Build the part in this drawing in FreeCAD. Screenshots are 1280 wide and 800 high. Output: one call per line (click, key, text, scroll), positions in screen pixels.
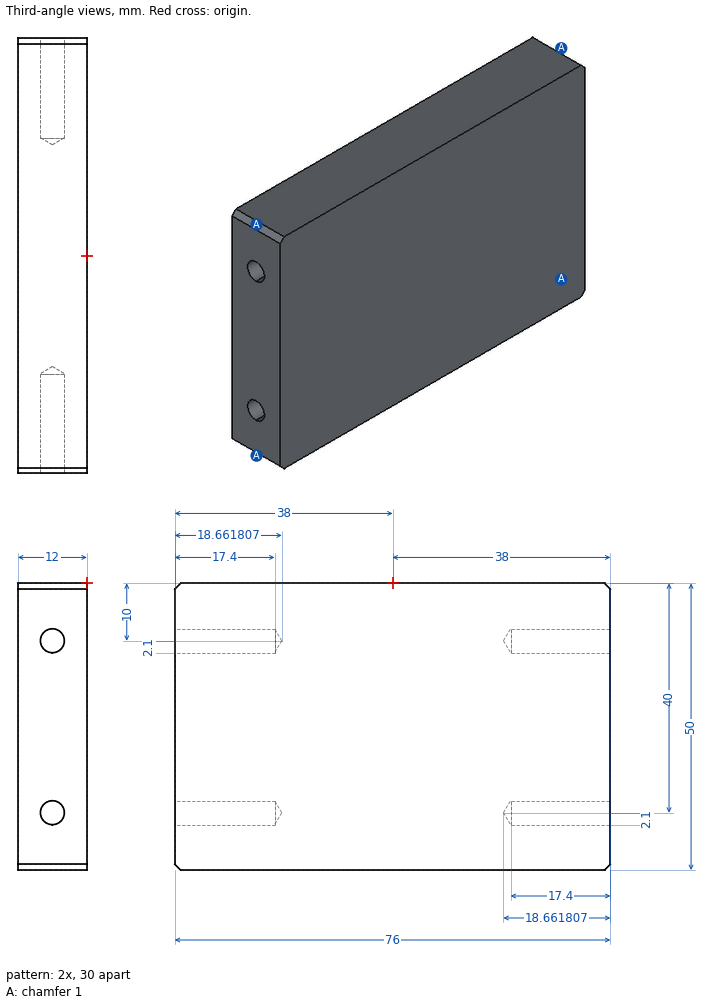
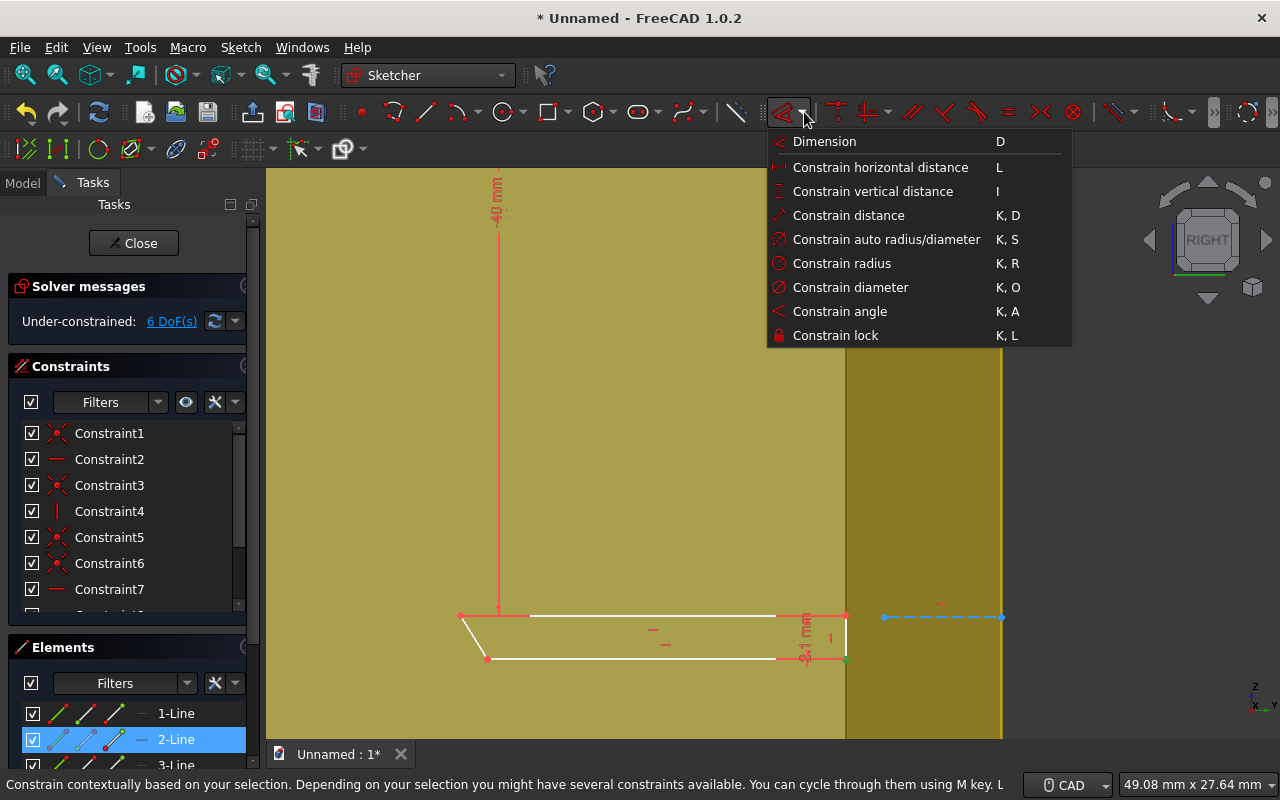
click(920, 167)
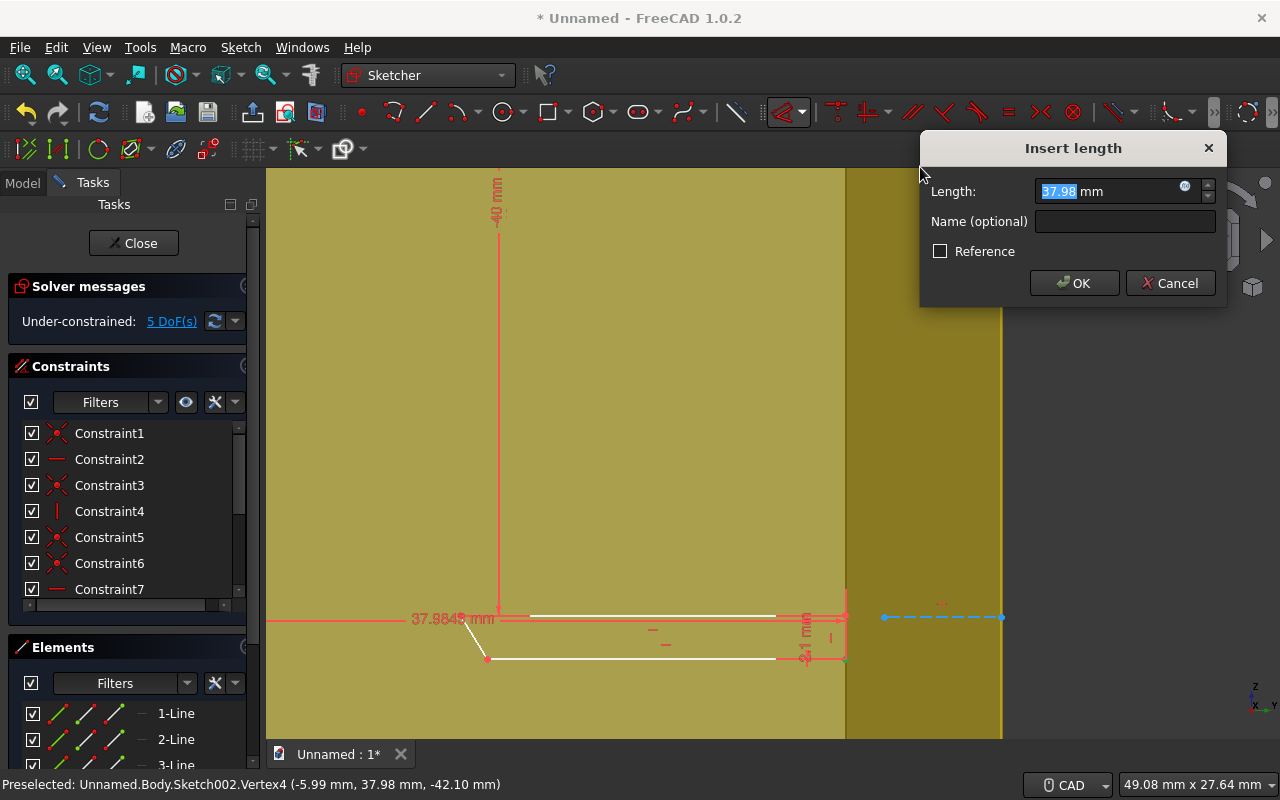
text(38)
key(Return)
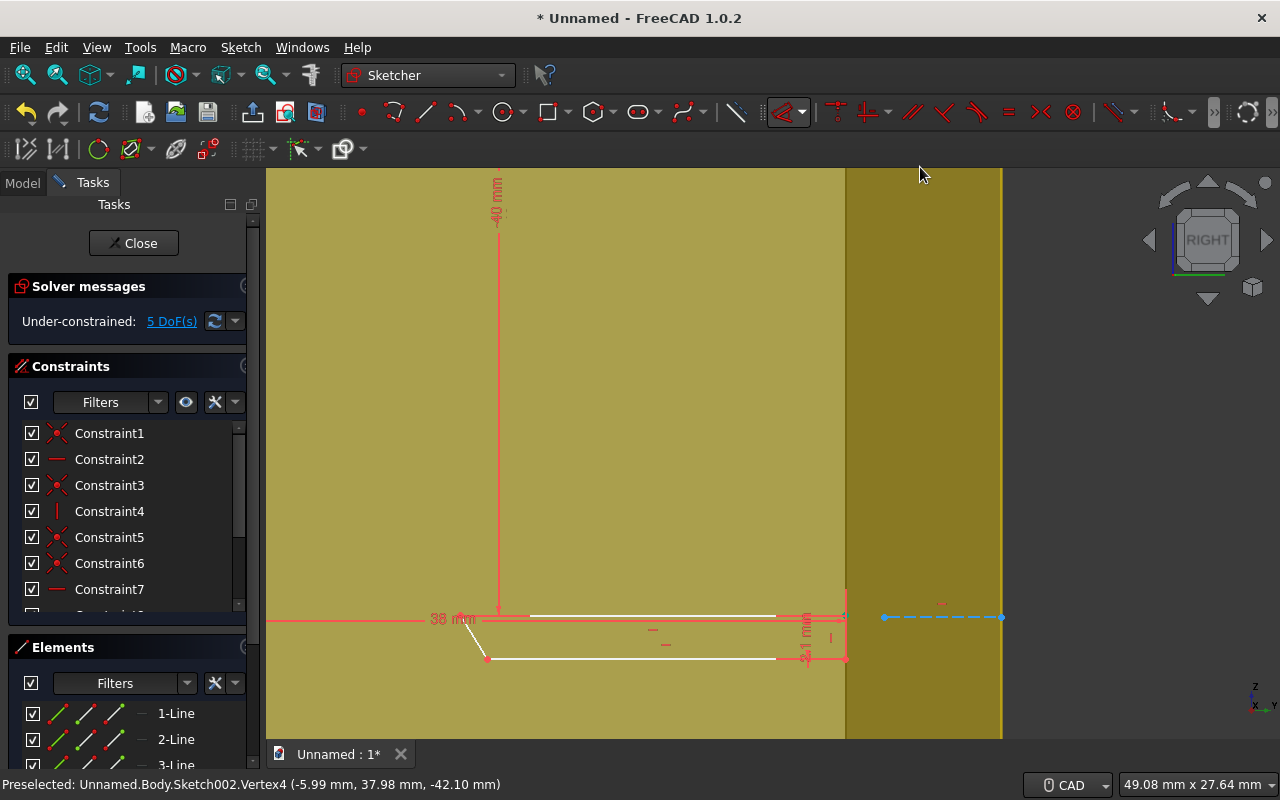
click(885, 617)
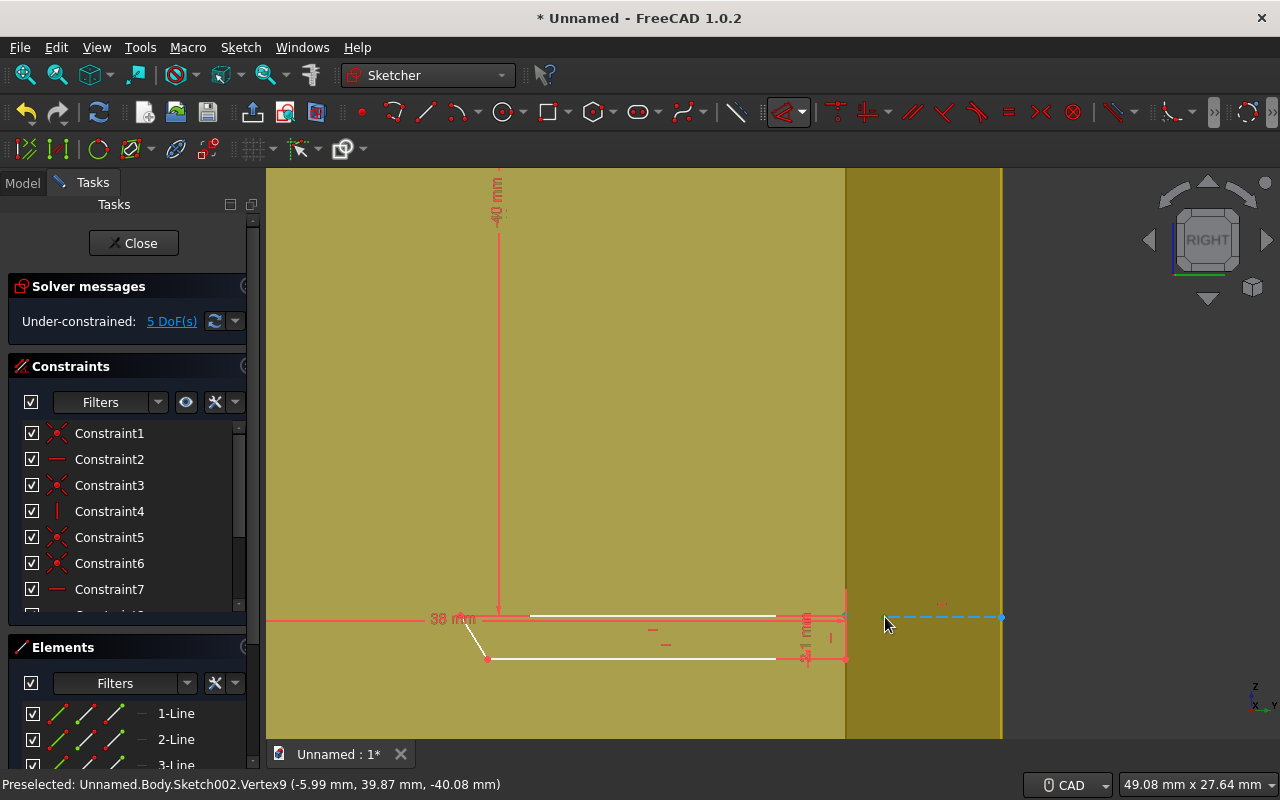
click(804, 112)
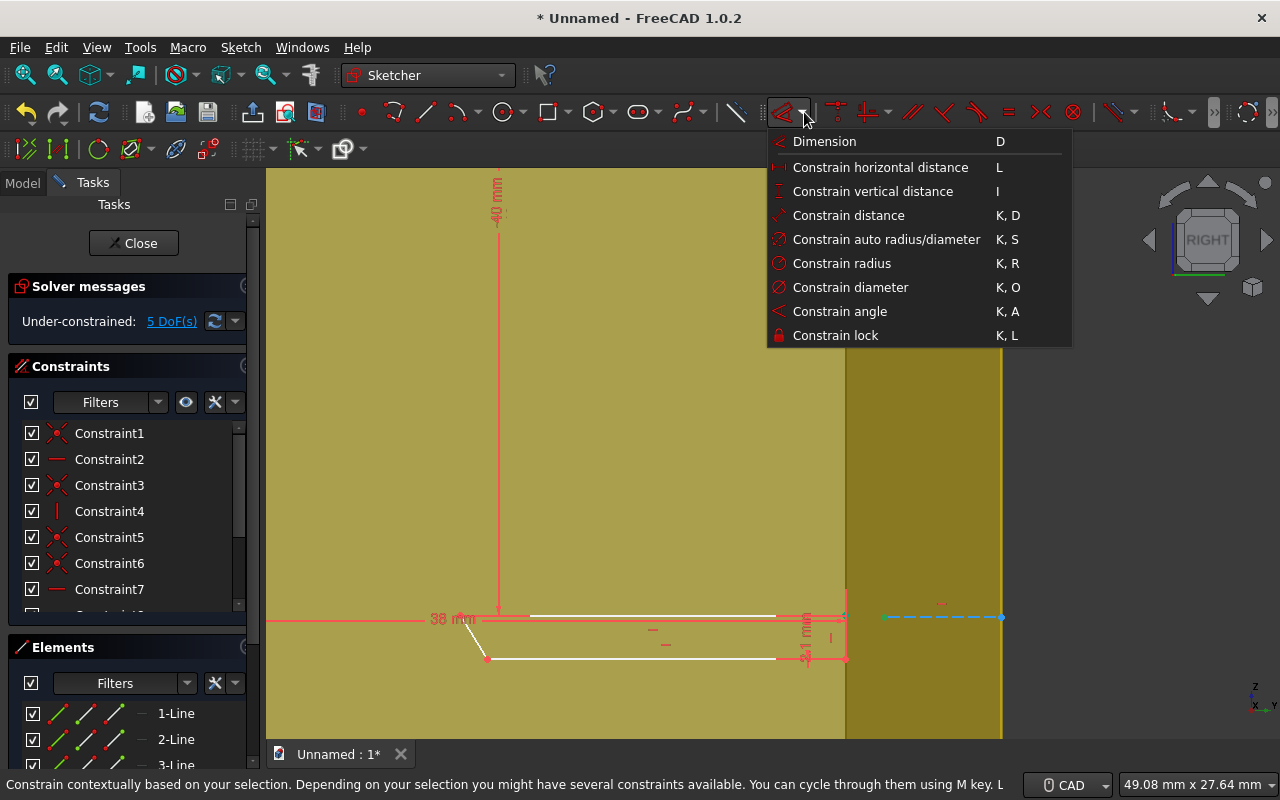
click(920, 191)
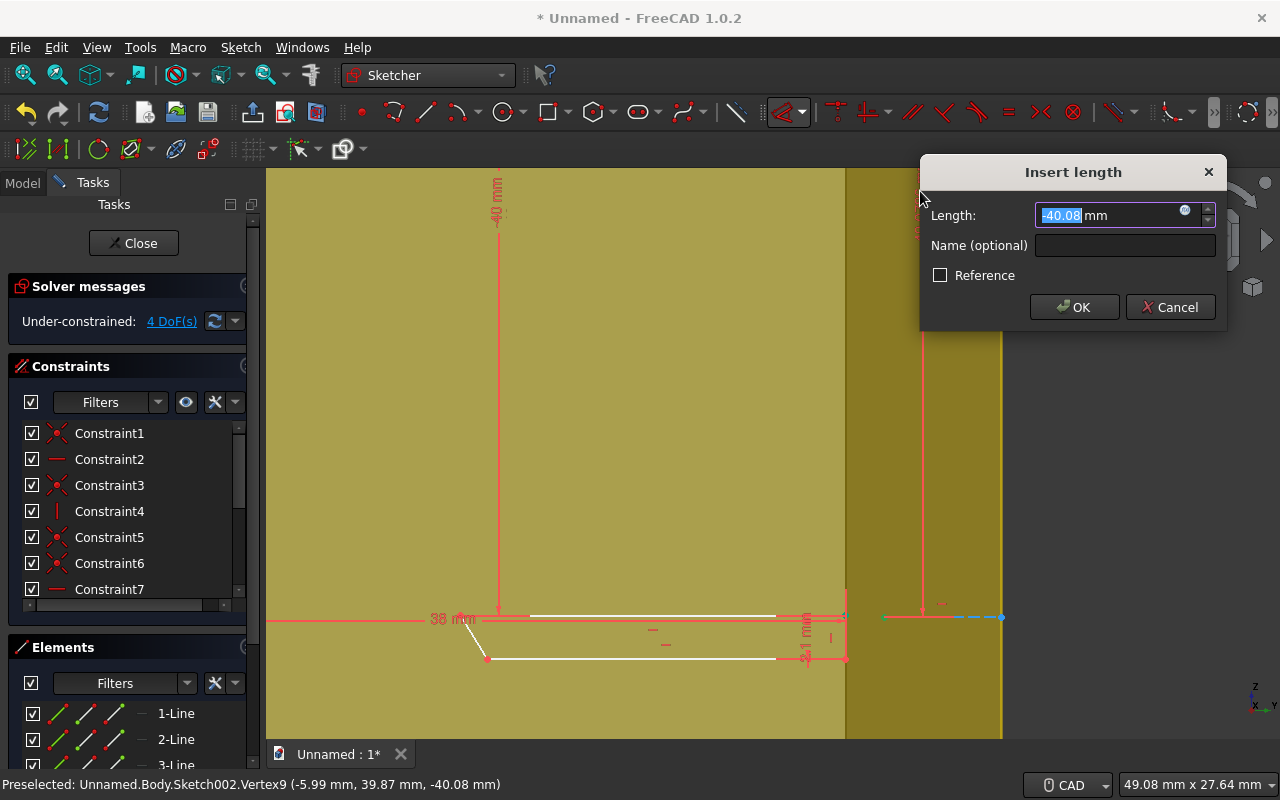
text(-40)
key(Return)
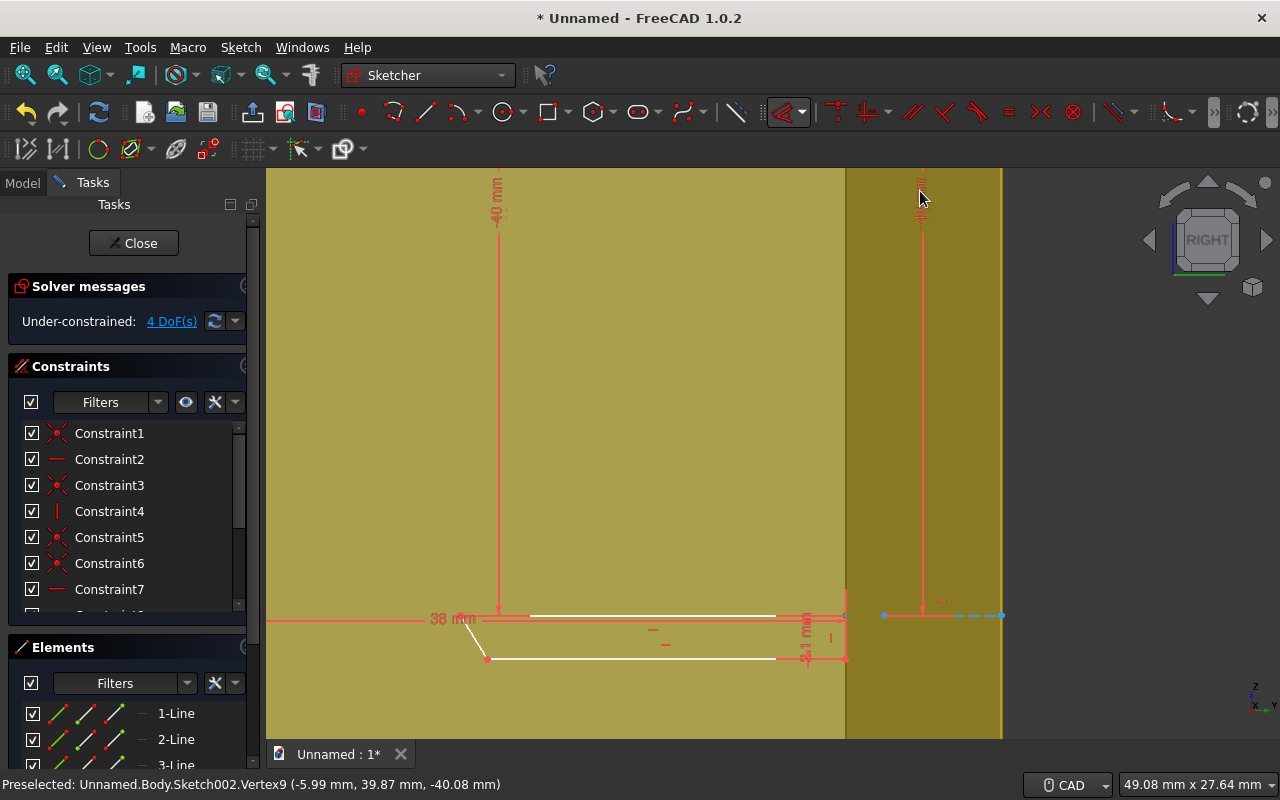
click(595, 659)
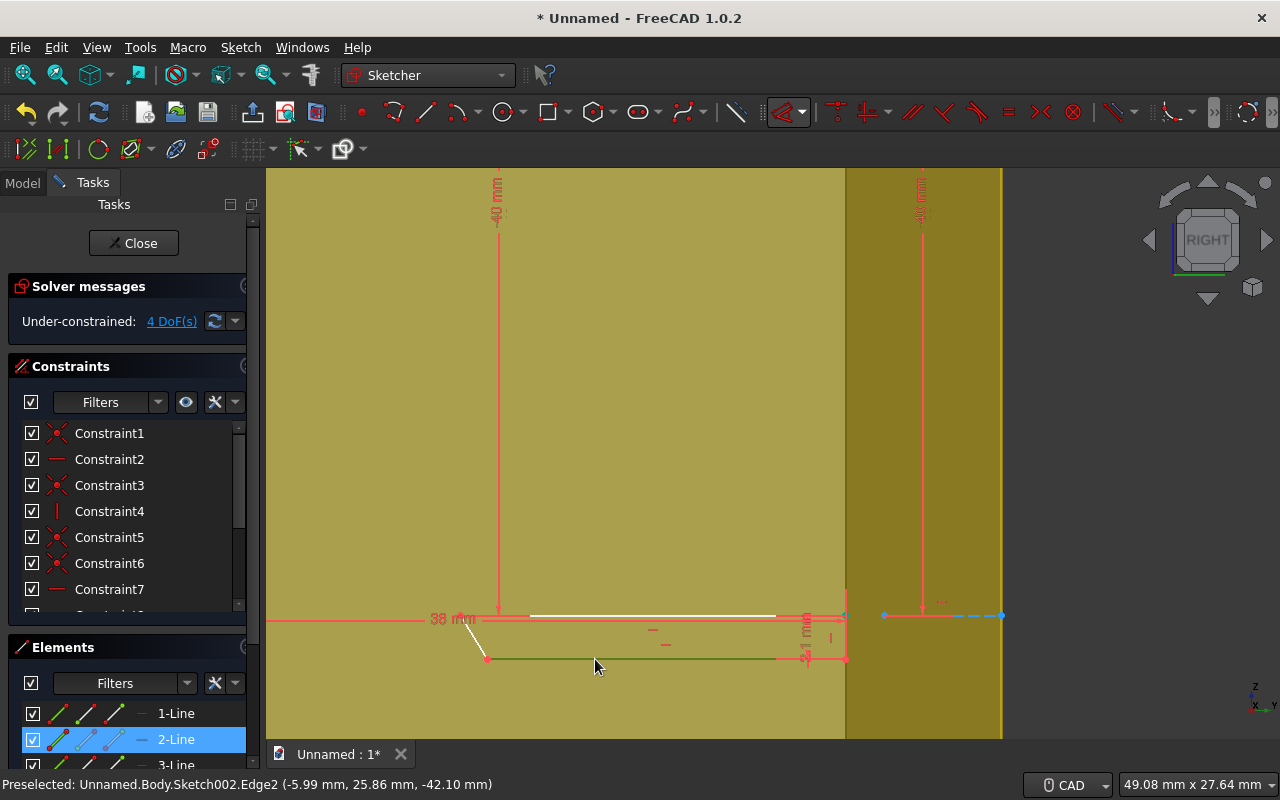
click(804, 112)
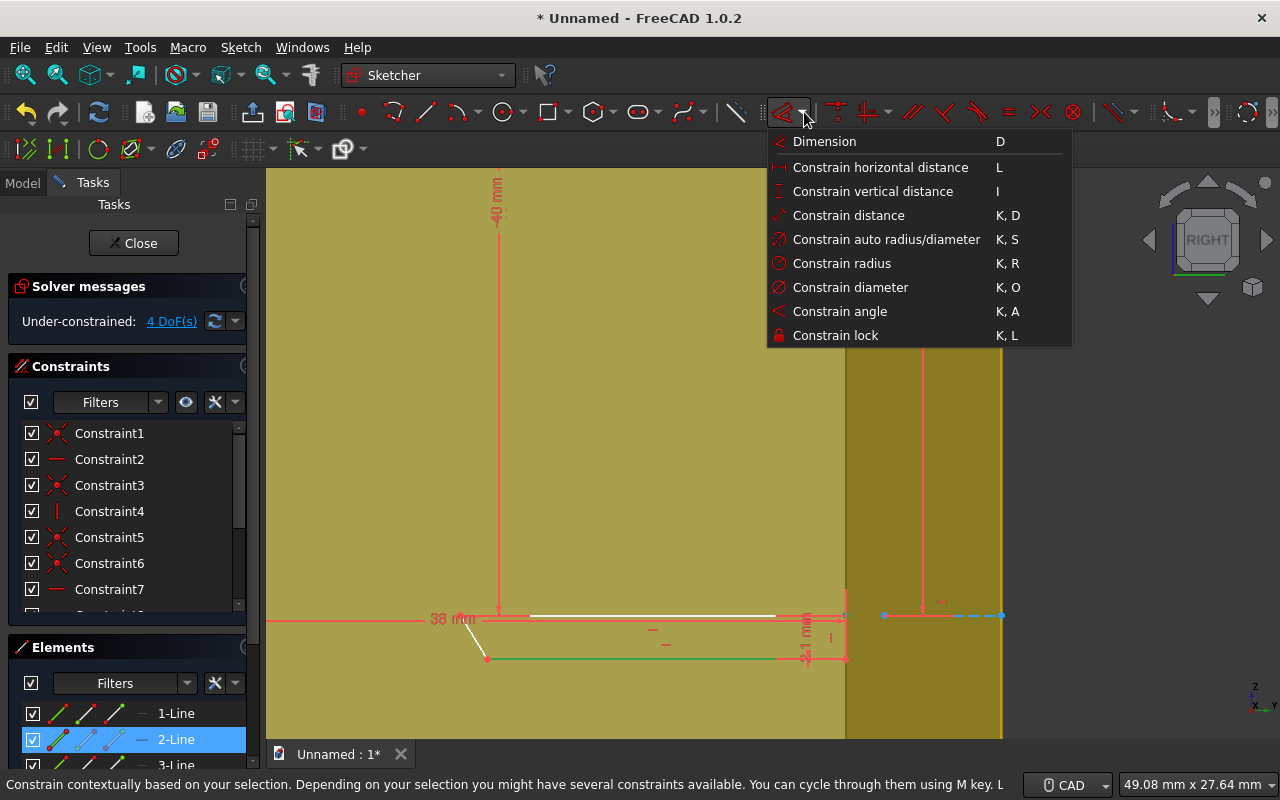
click(920, 167)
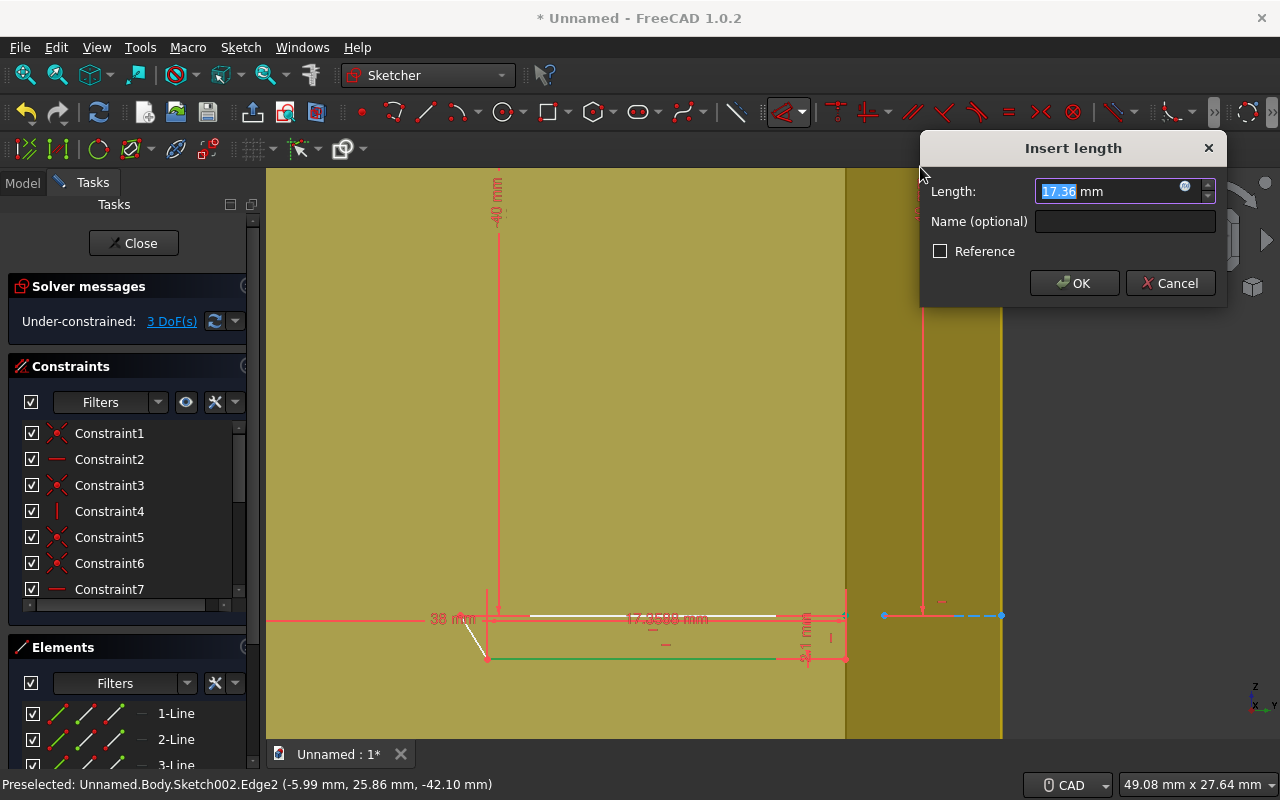
text(17.4)
key(Return)